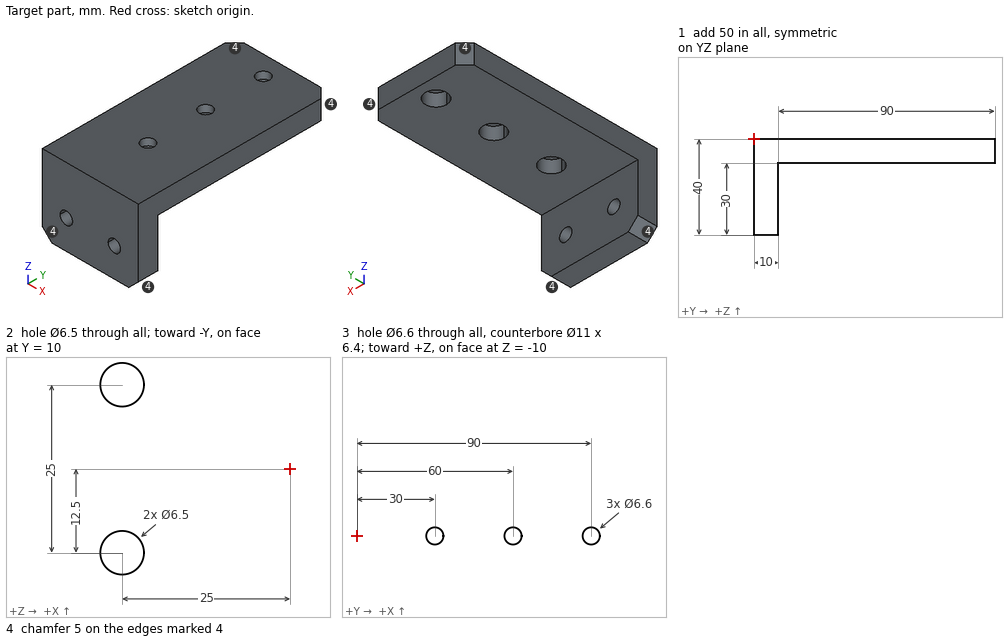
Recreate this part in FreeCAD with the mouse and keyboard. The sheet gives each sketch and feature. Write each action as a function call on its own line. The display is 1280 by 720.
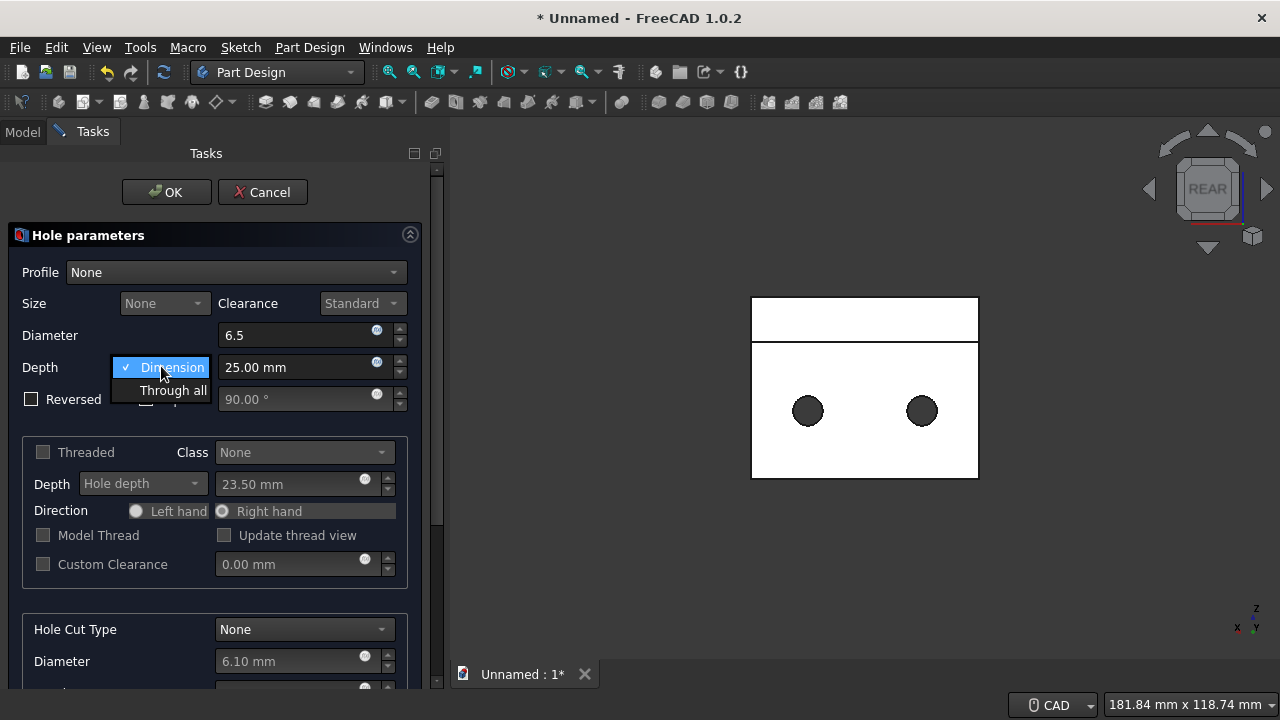
click(160, 390)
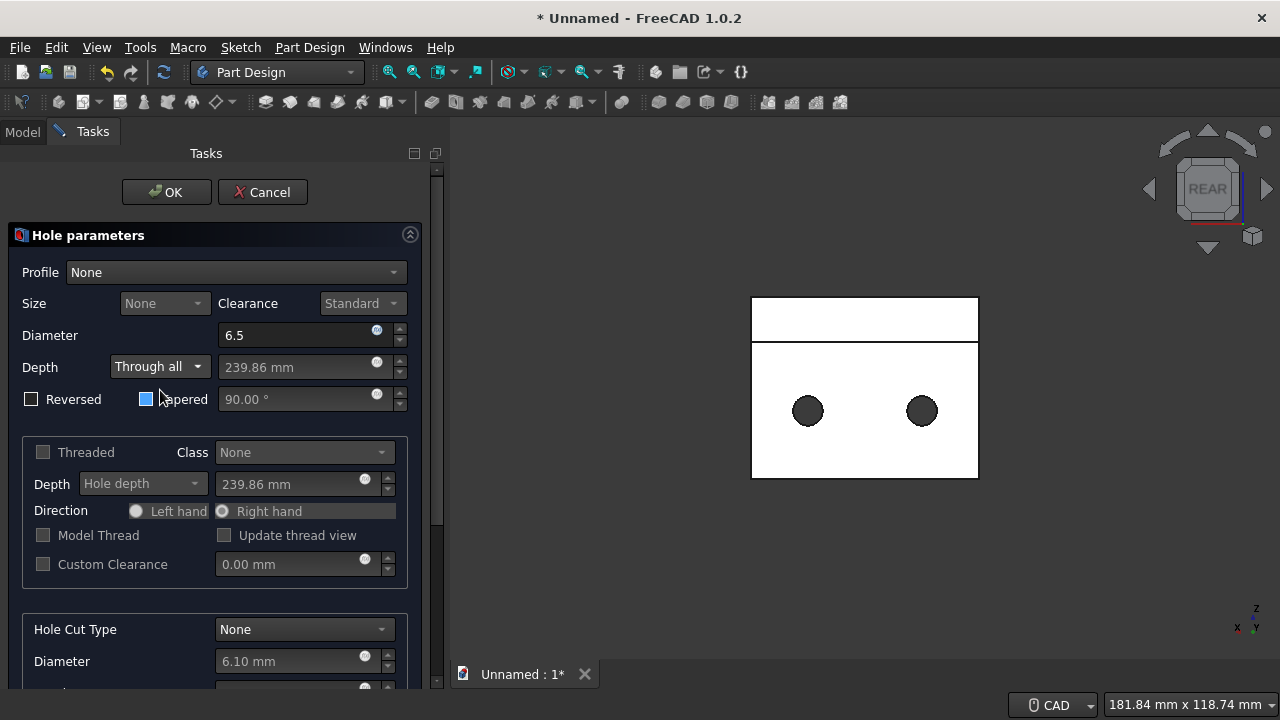
click(167, 192)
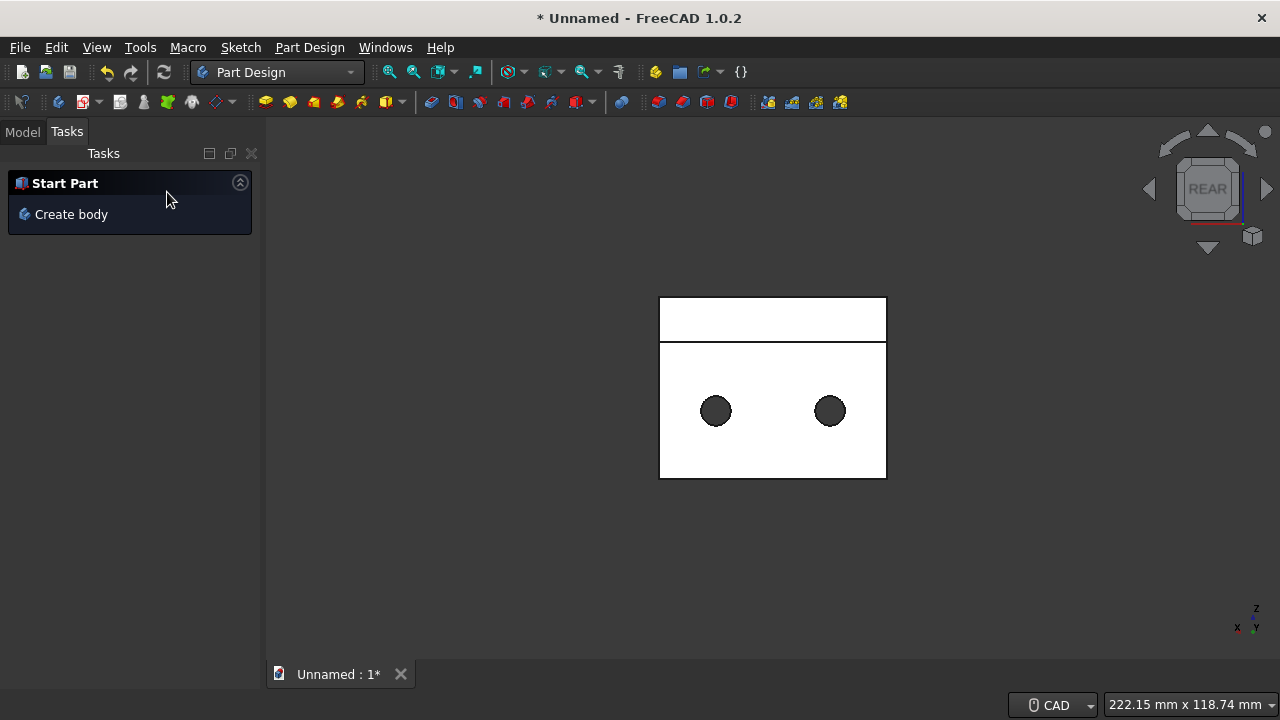
click(390, 72)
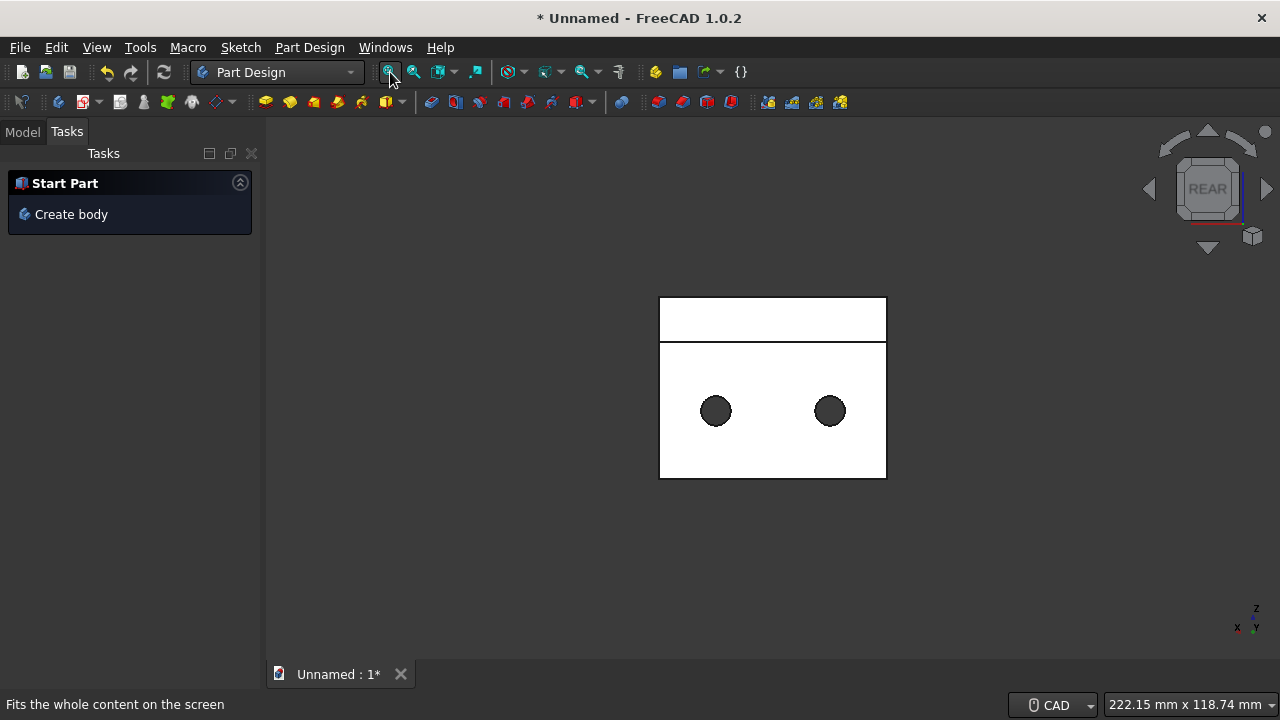
key(5)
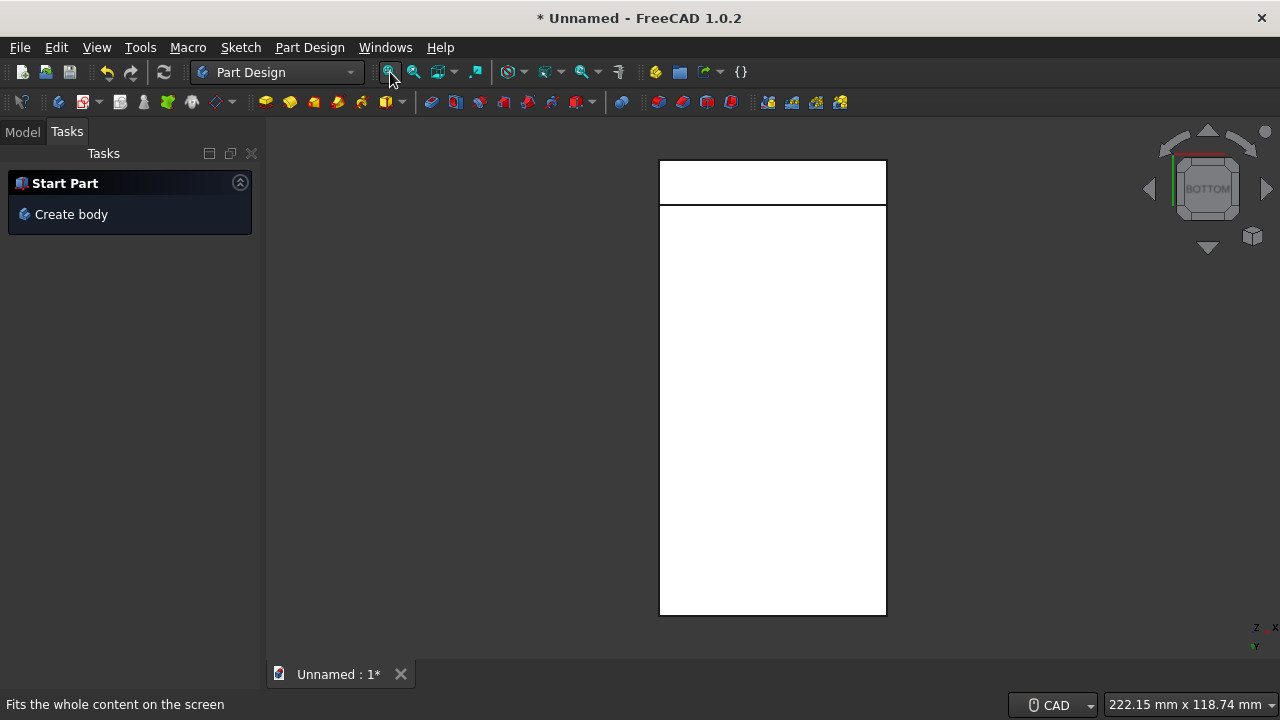
click(773, 469)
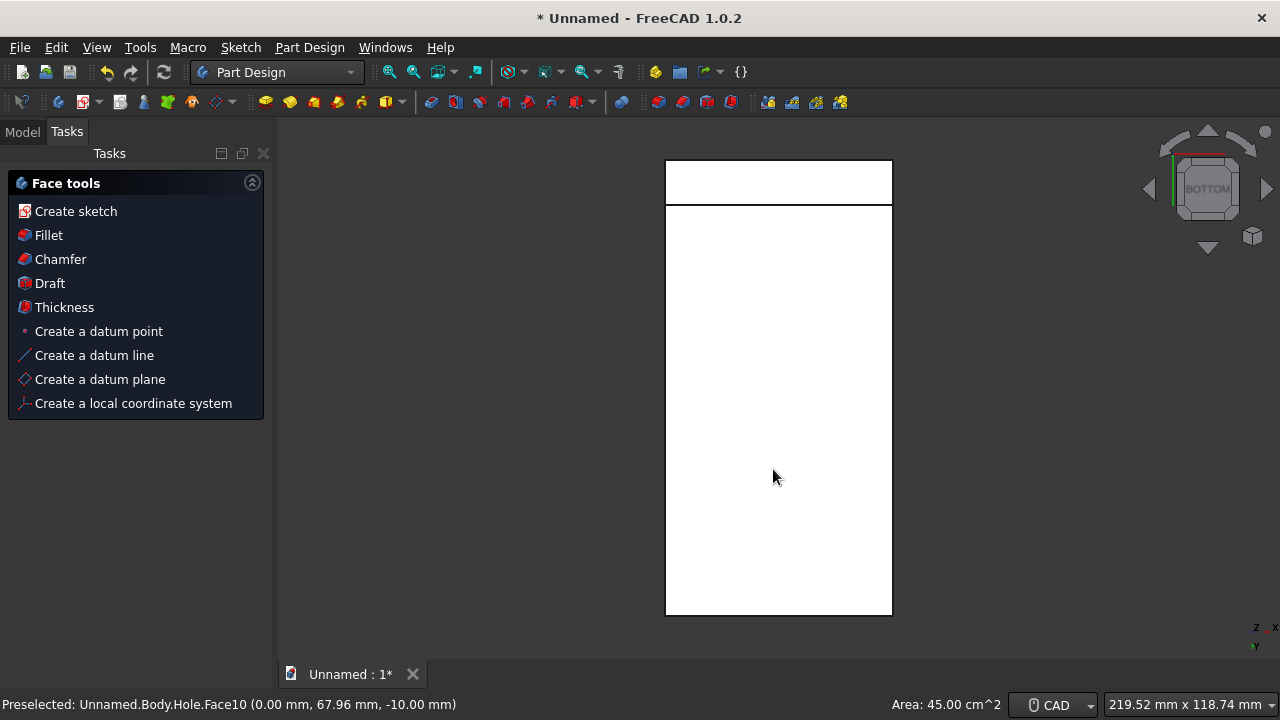
click(84, 102)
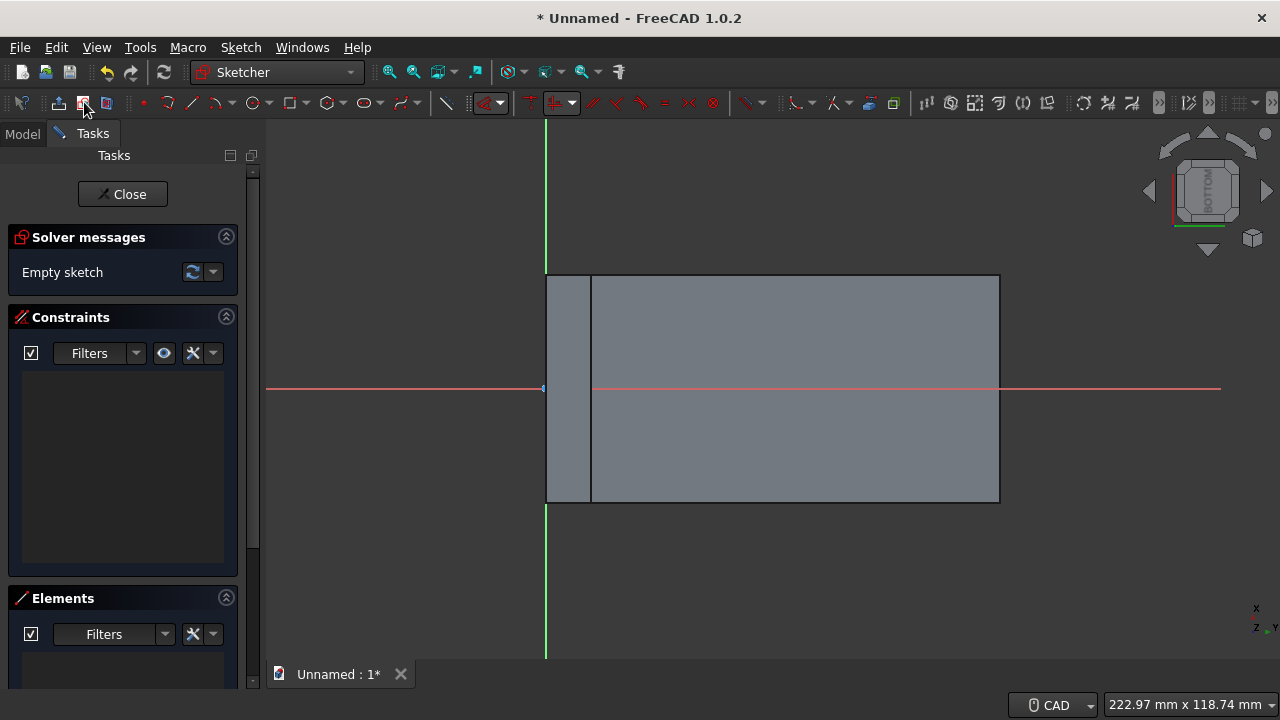
click(108, 104)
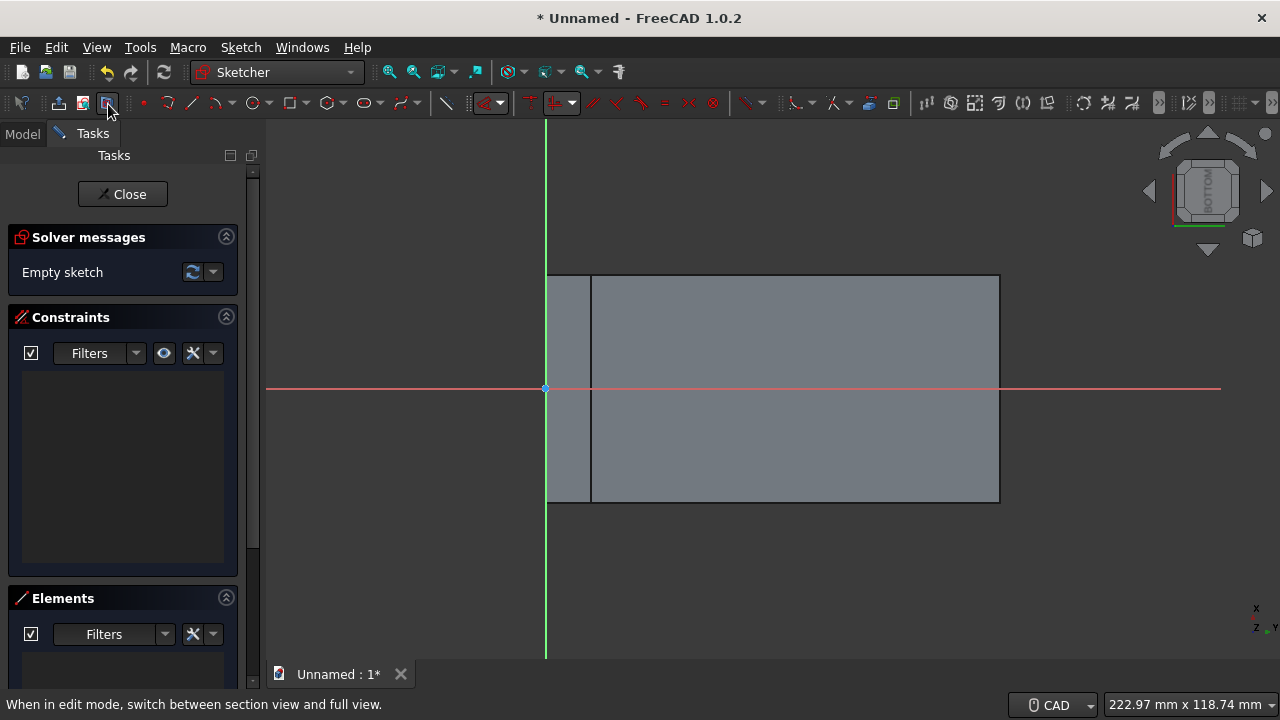
scroll(866, 389, up, 2)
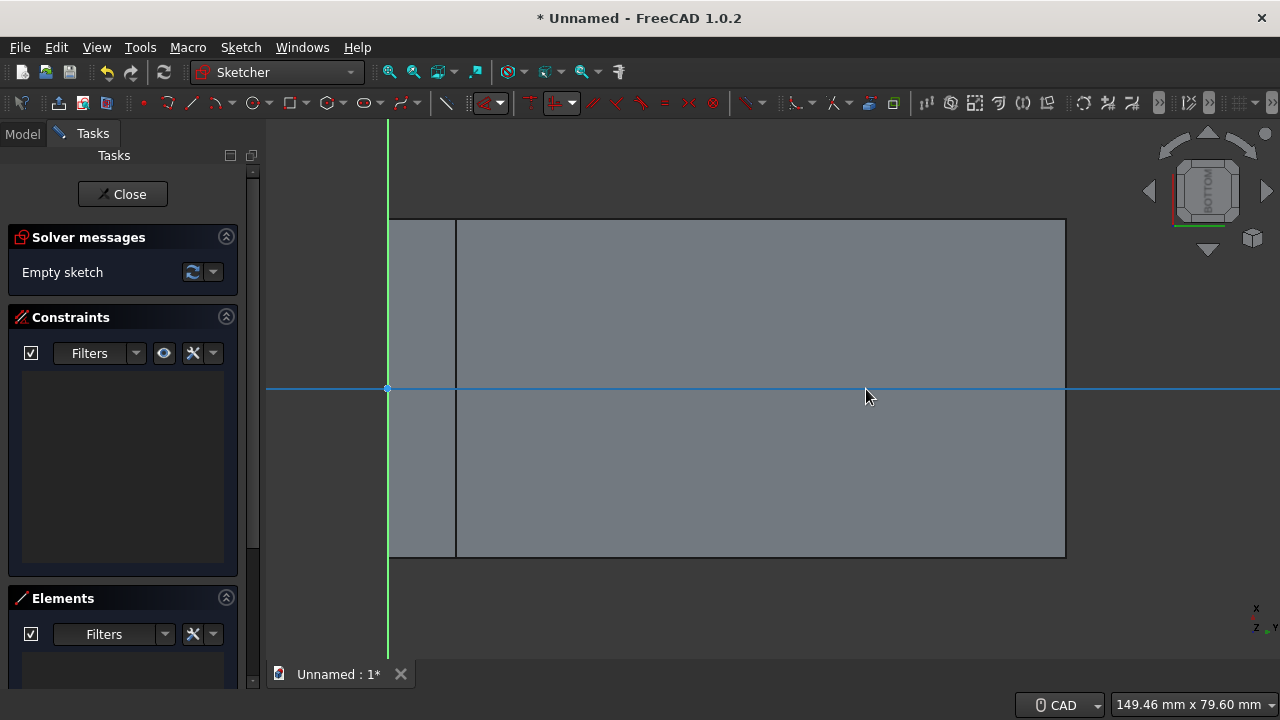
click(254, 104)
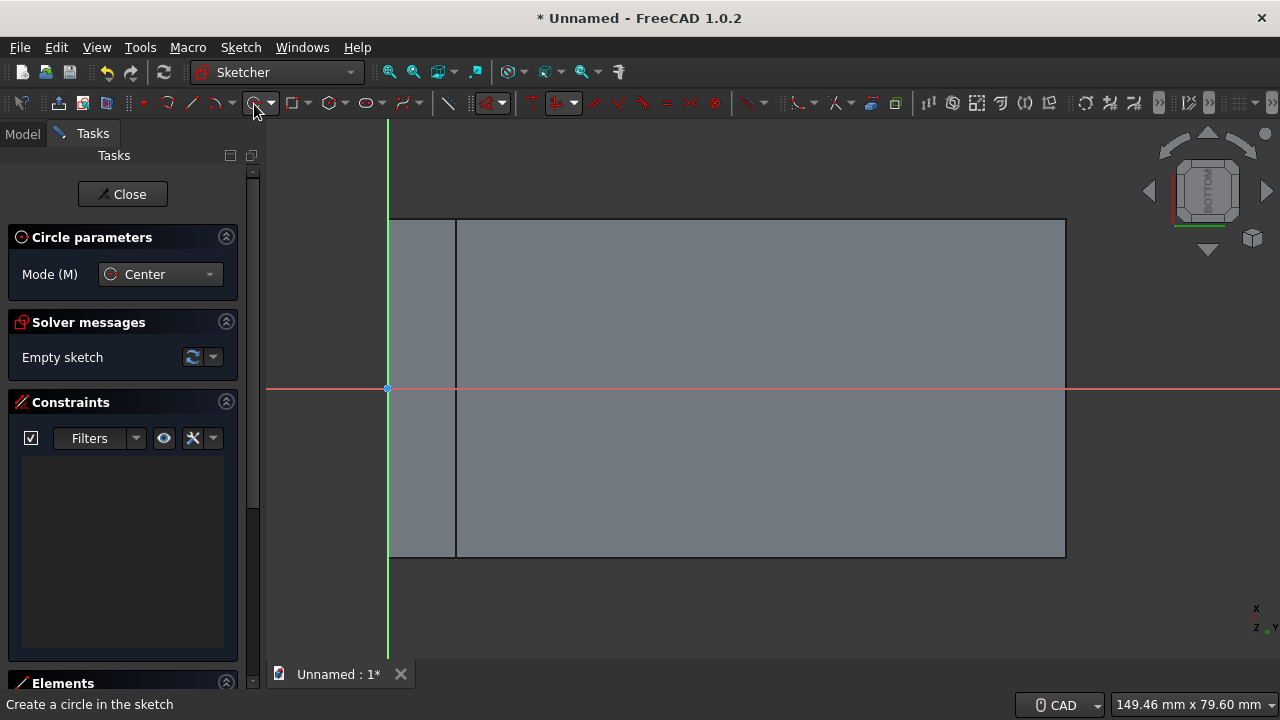
click(998, 389)
click(1014, 373)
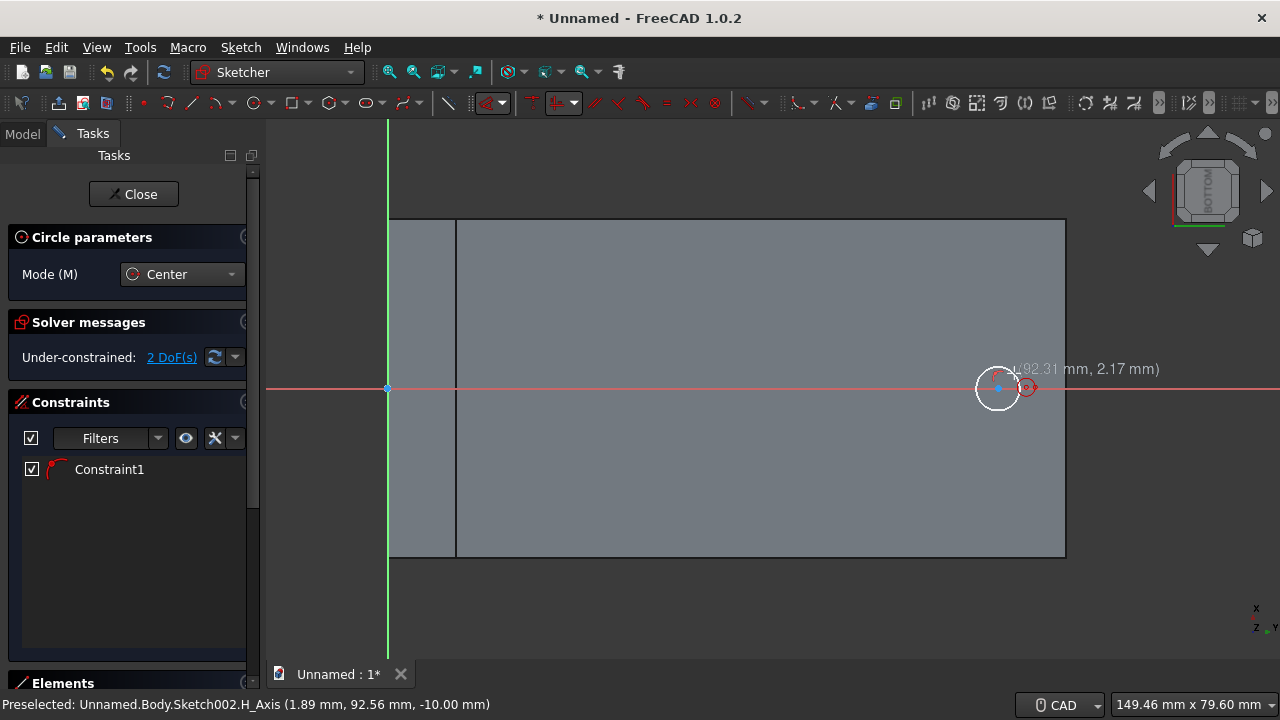
click(795, 389)
click(811, 373)